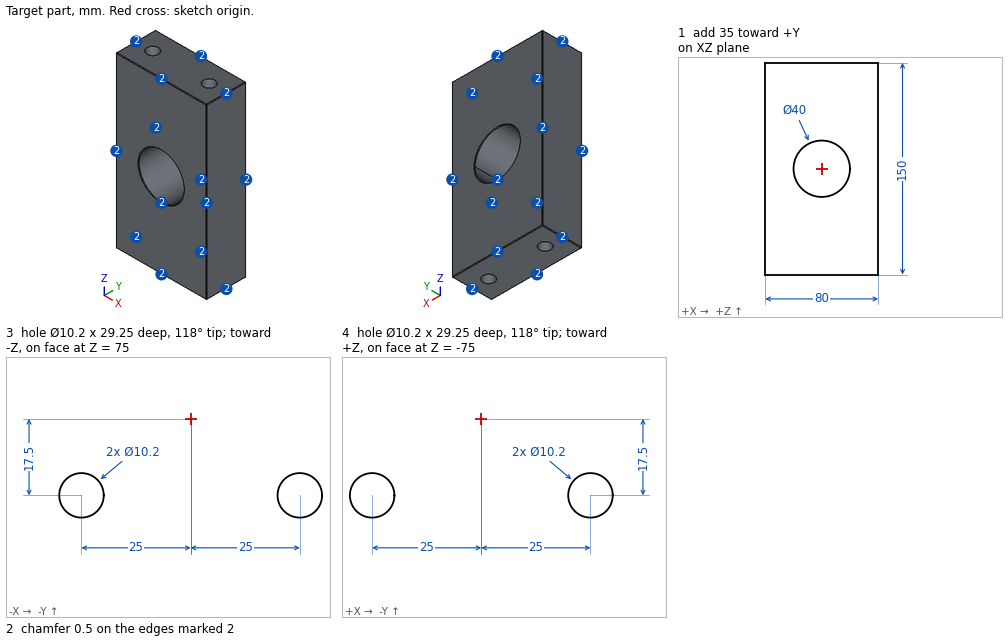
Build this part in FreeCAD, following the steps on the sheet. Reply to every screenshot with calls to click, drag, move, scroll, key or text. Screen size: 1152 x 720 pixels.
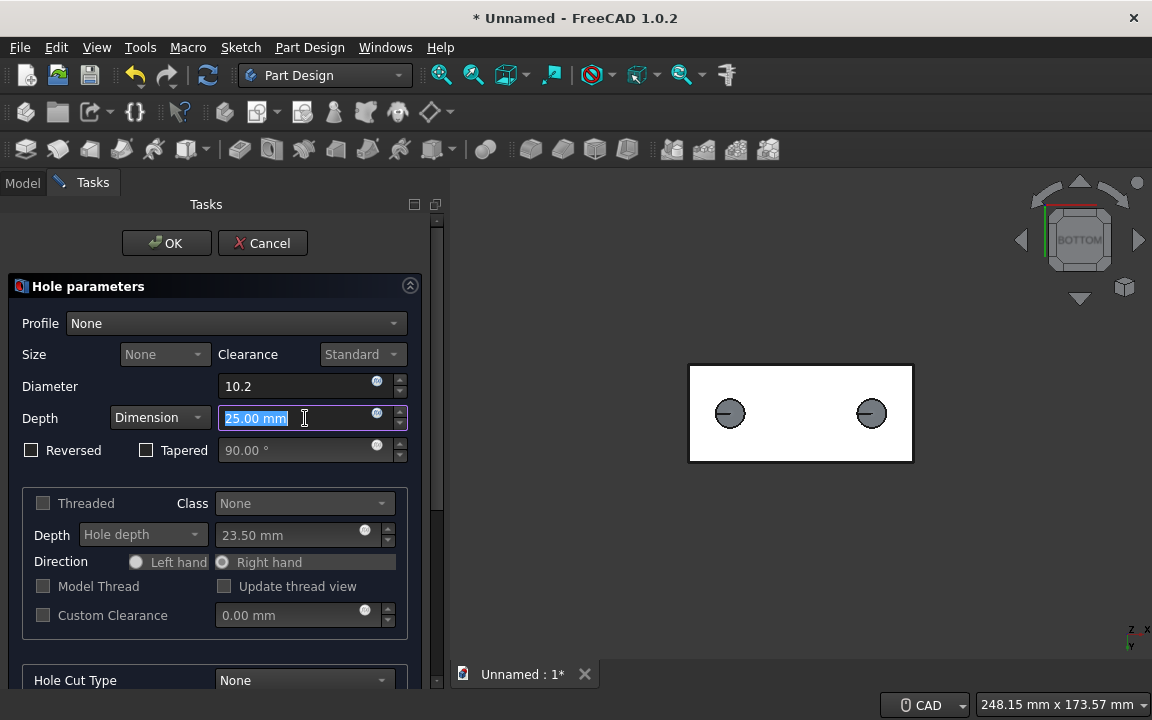
text(29.25)
key(Tab)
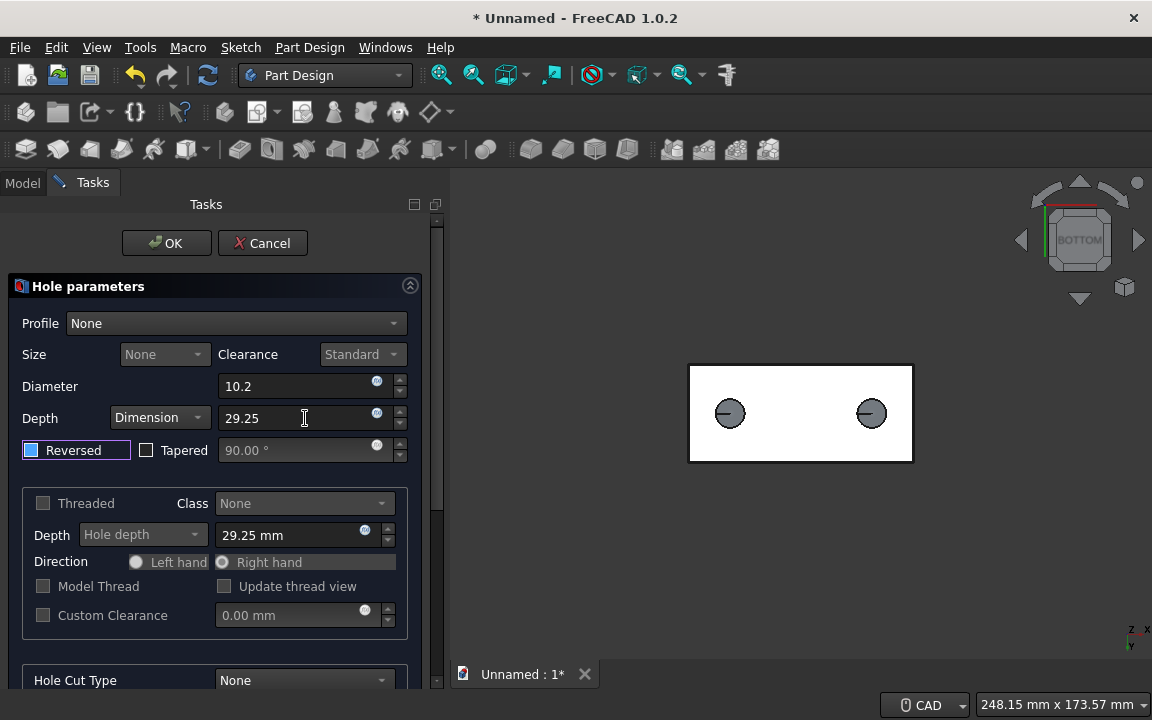
click(167, 243)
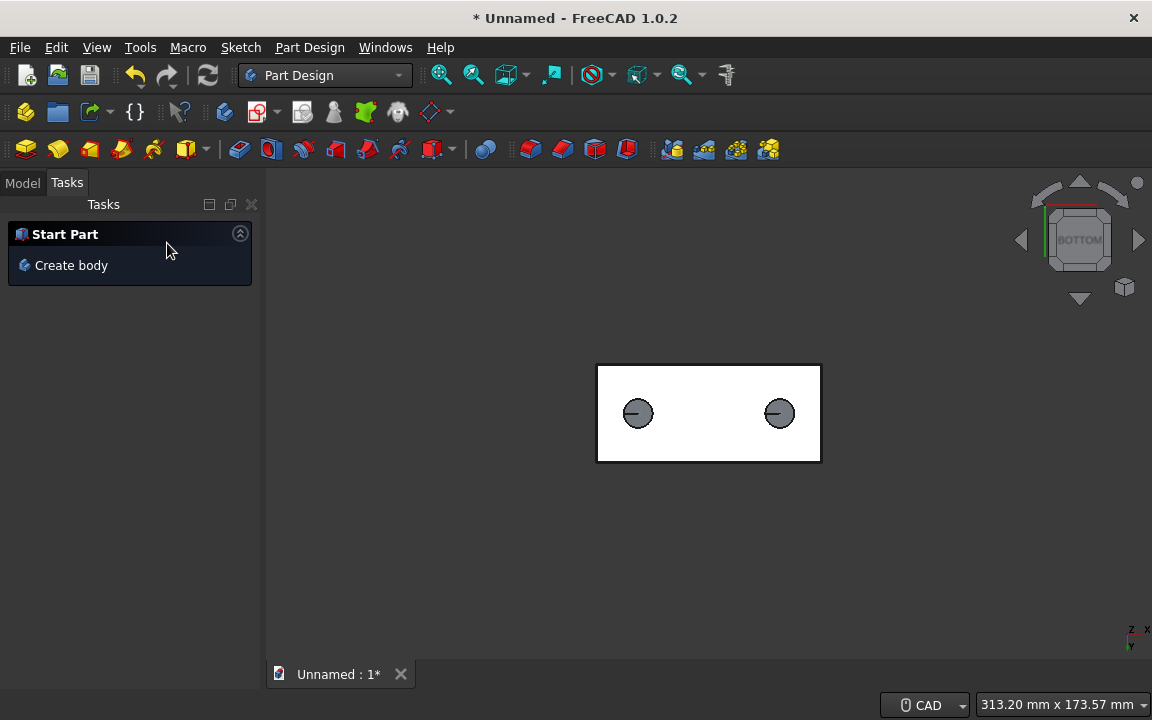
key(0)